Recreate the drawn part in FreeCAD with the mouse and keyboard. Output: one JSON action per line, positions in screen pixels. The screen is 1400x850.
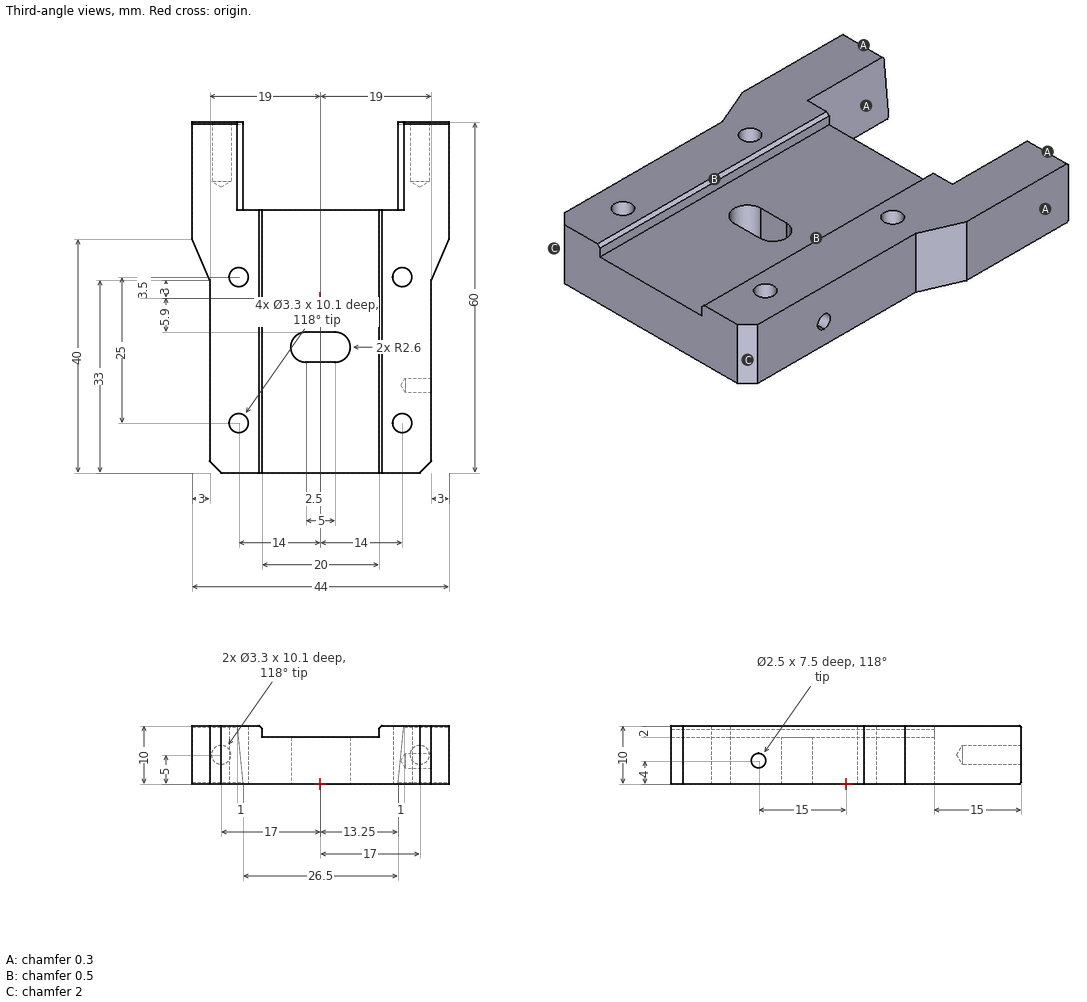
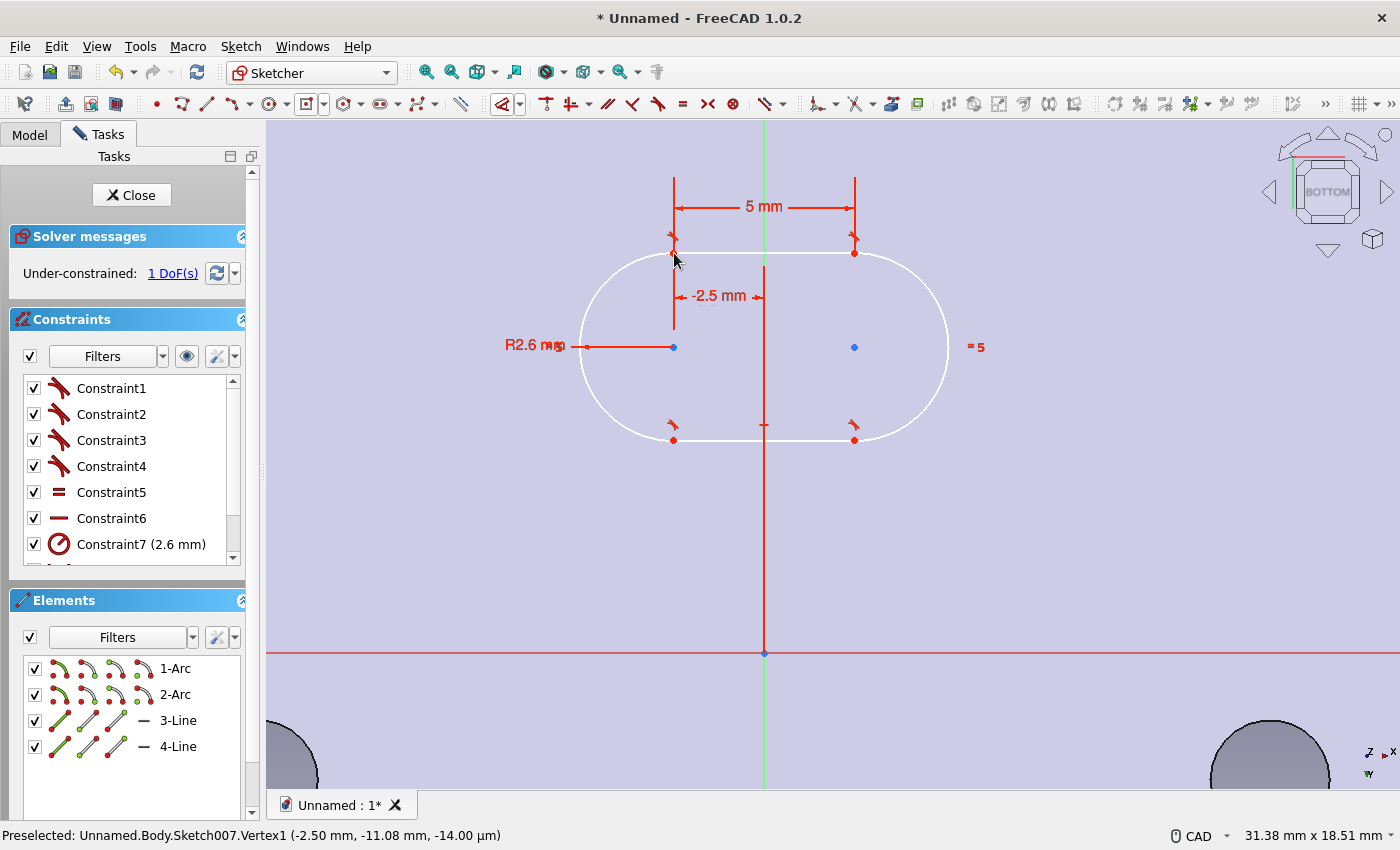
{"action": "left_click", "coordinate": [674, 441]}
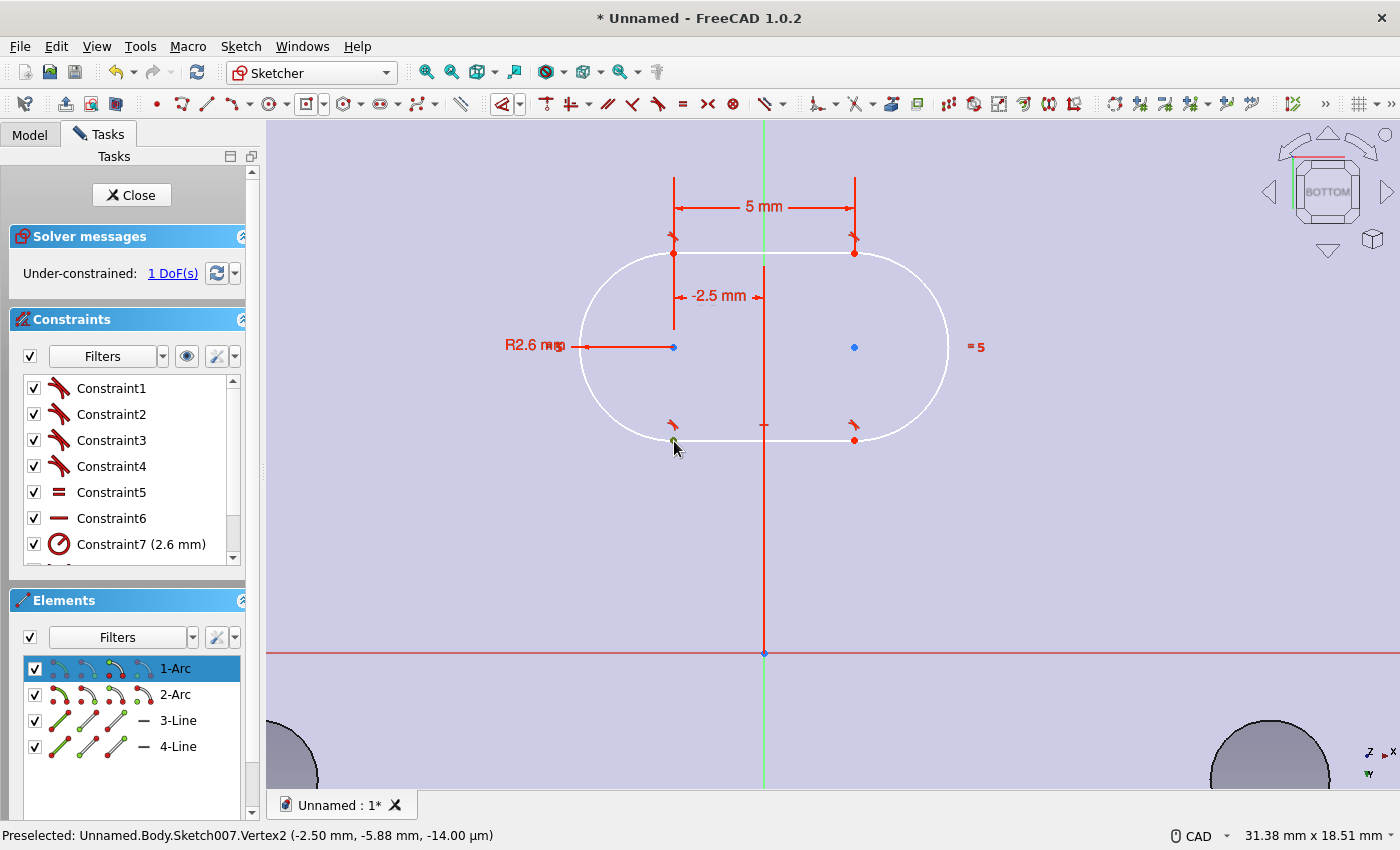
{"action": "left_click", "coordinate": [520, 104]}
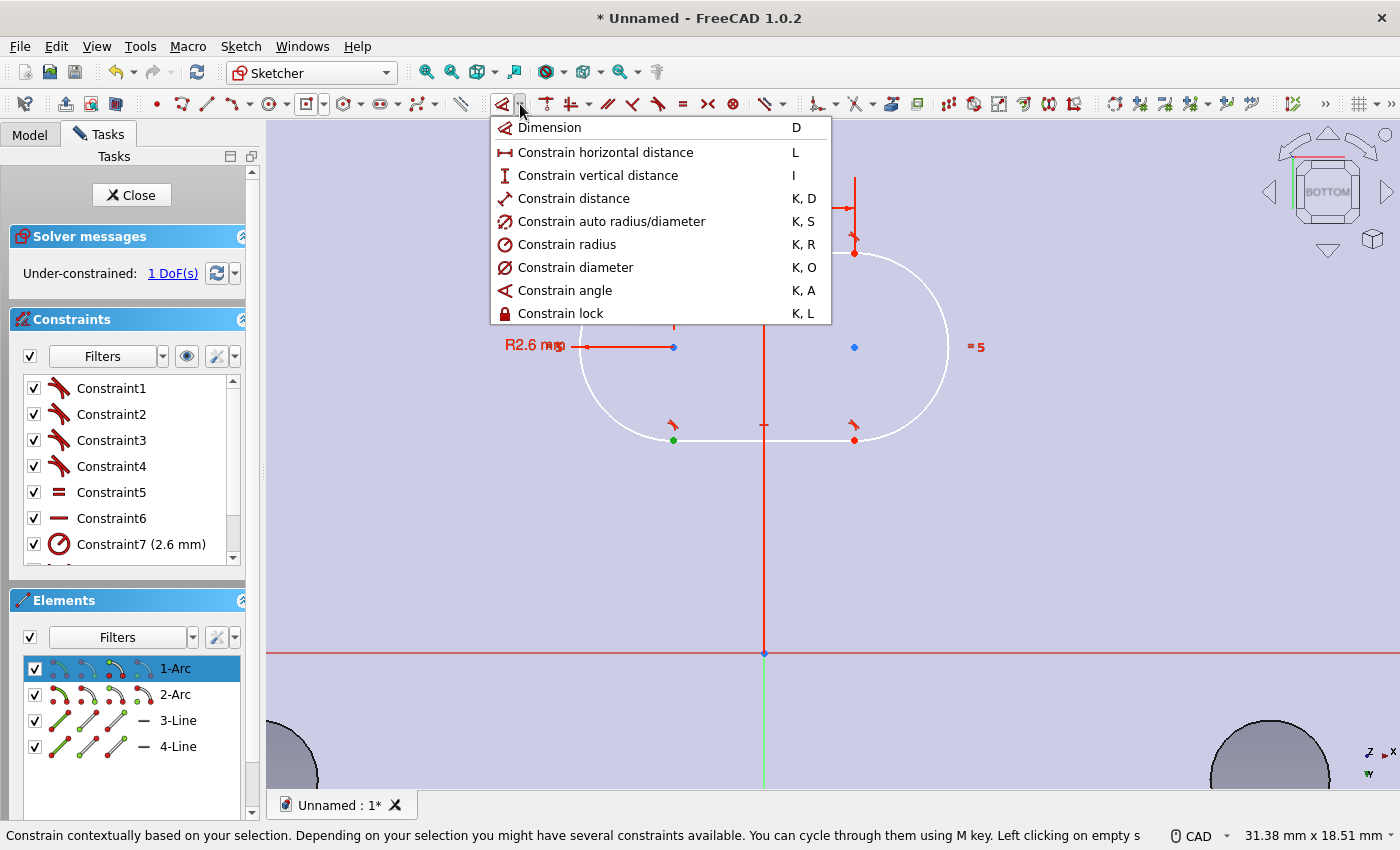
{"action": "left_click", "coordinate": [661, 176]}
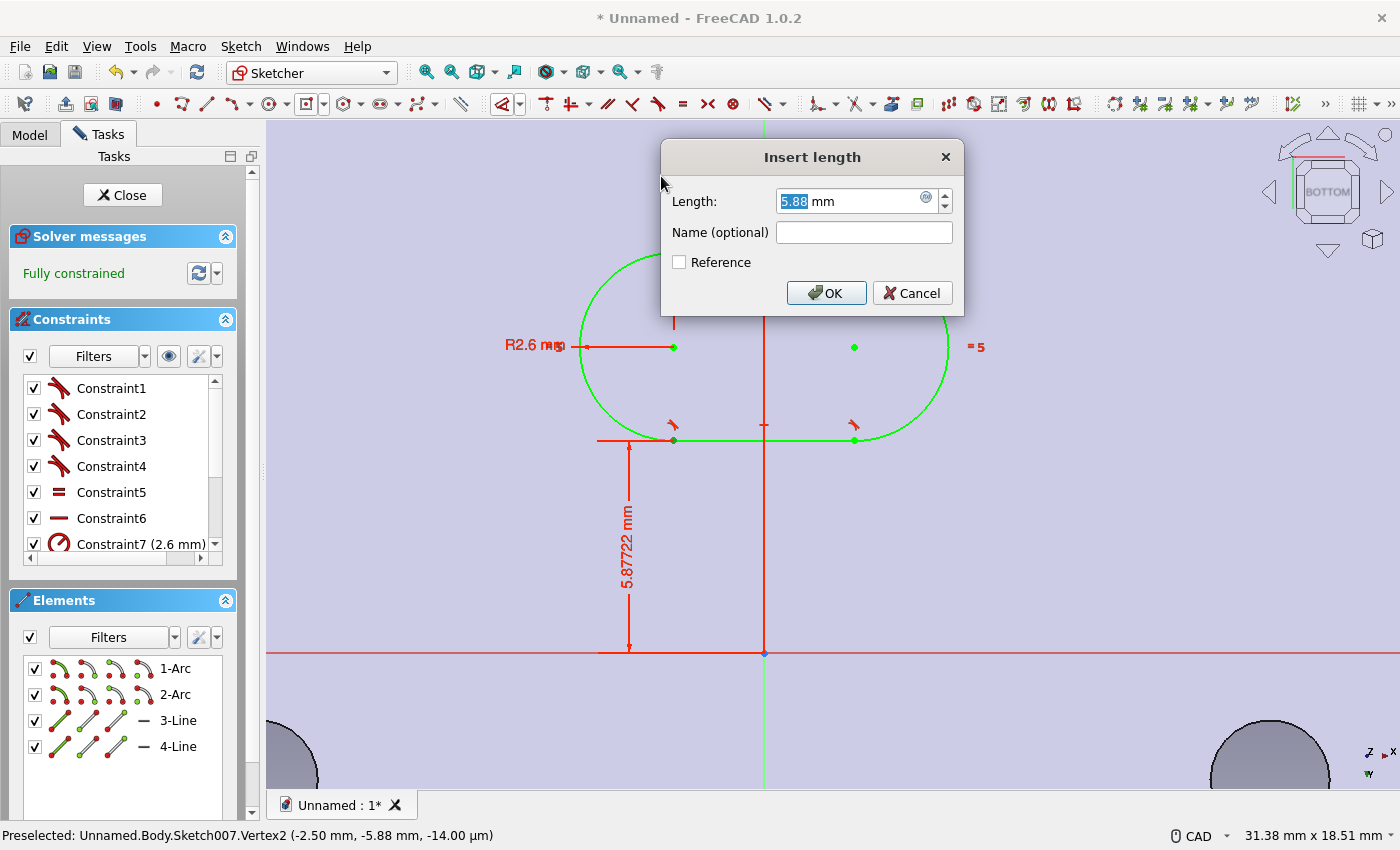
{"action": "type", "text": "5.9"}
{"action": "key", "text": "Return"}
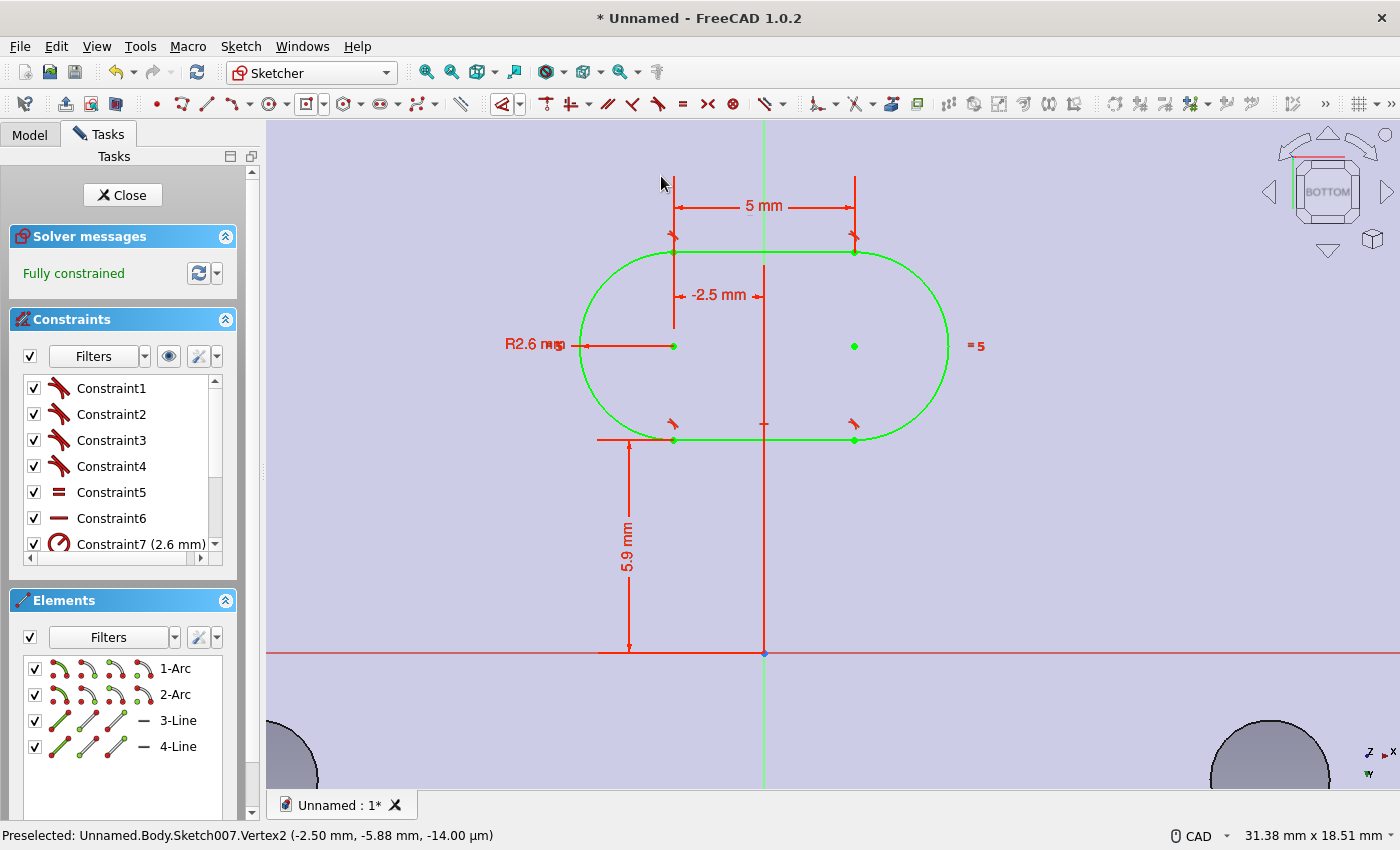
{"action": "left_click", "coordinate": [123, 195]}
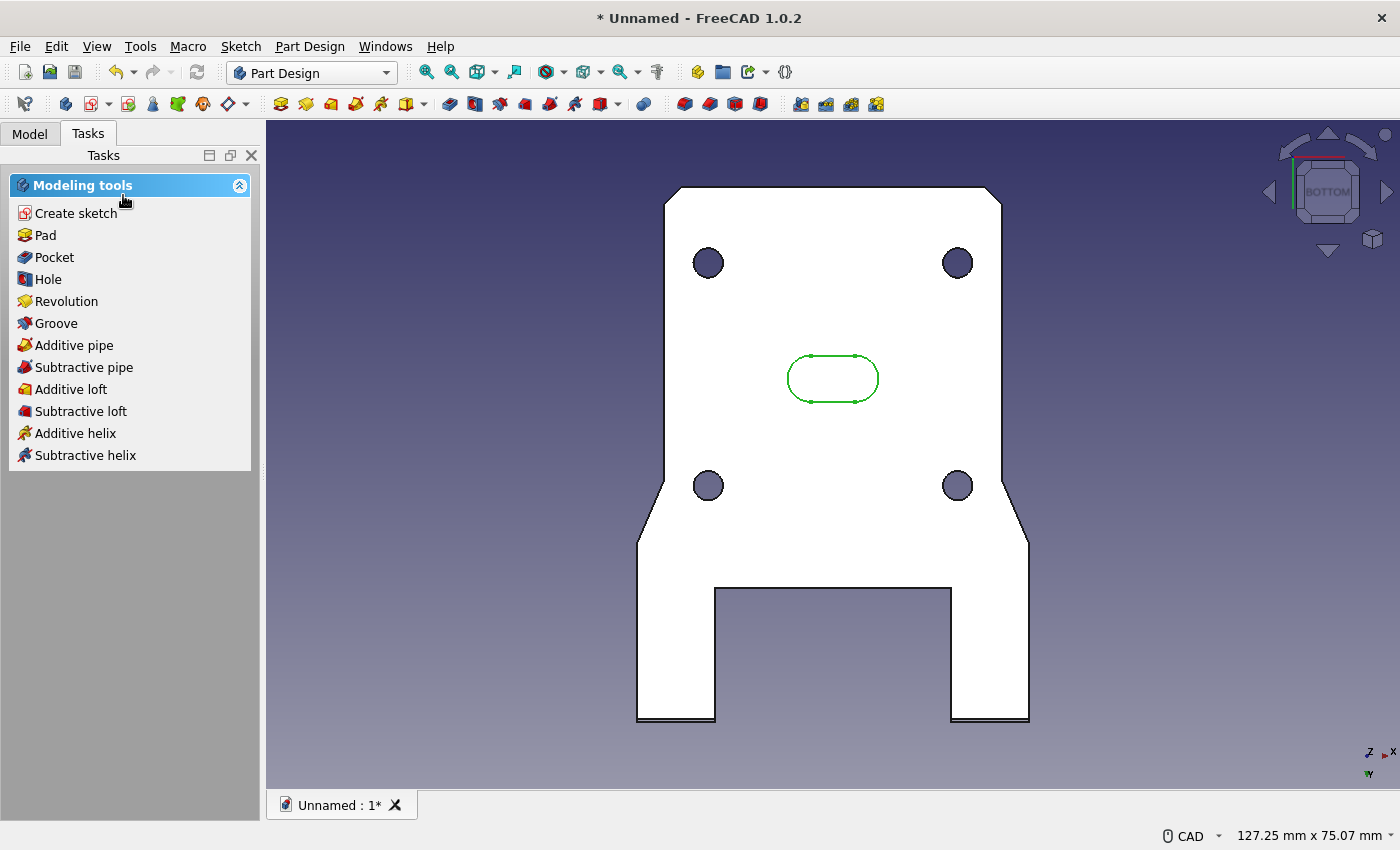
{"action": "left_click", "coordinate": [450, 104]}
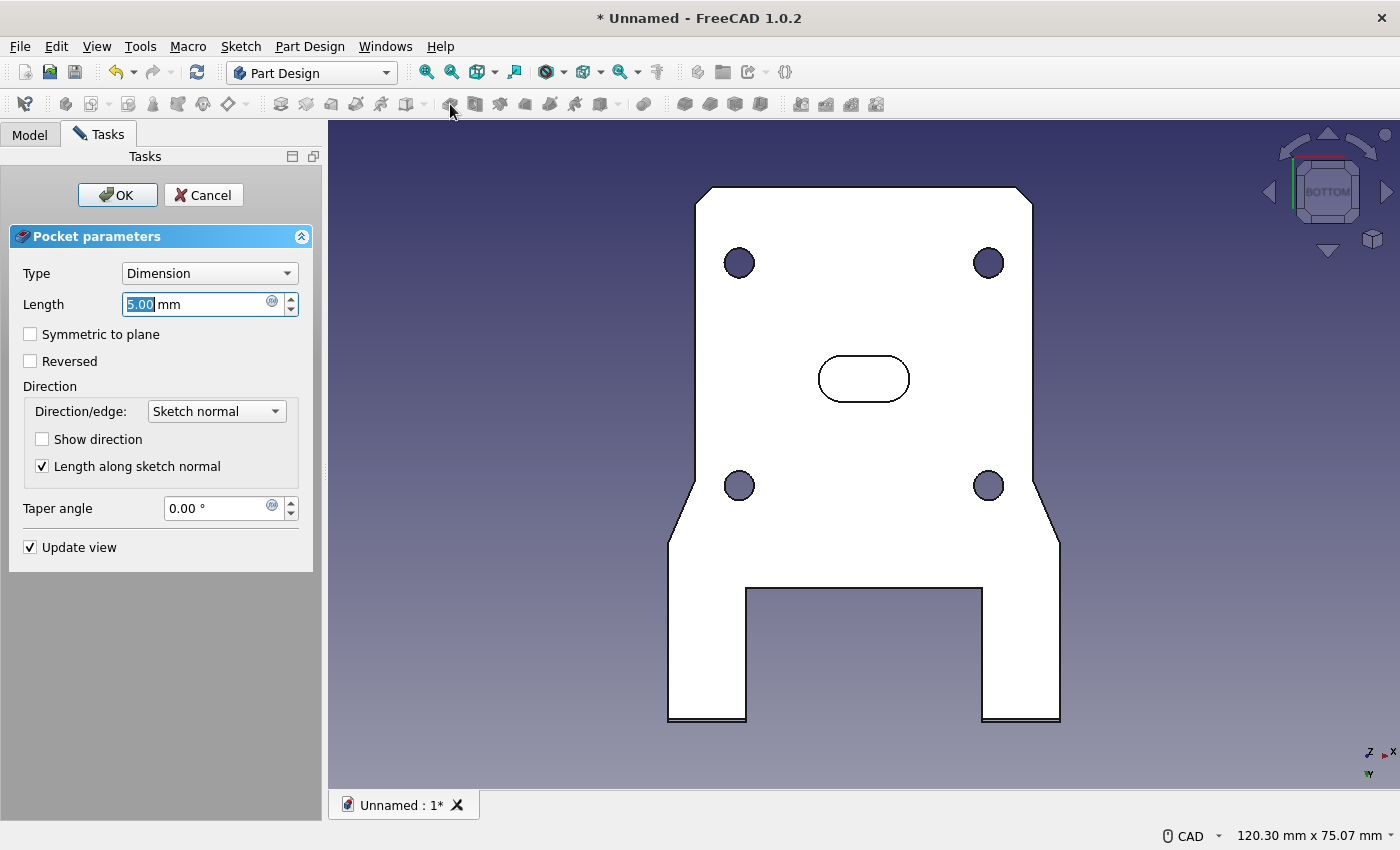
{"action": "left_click", "coordinate": [210, 274]}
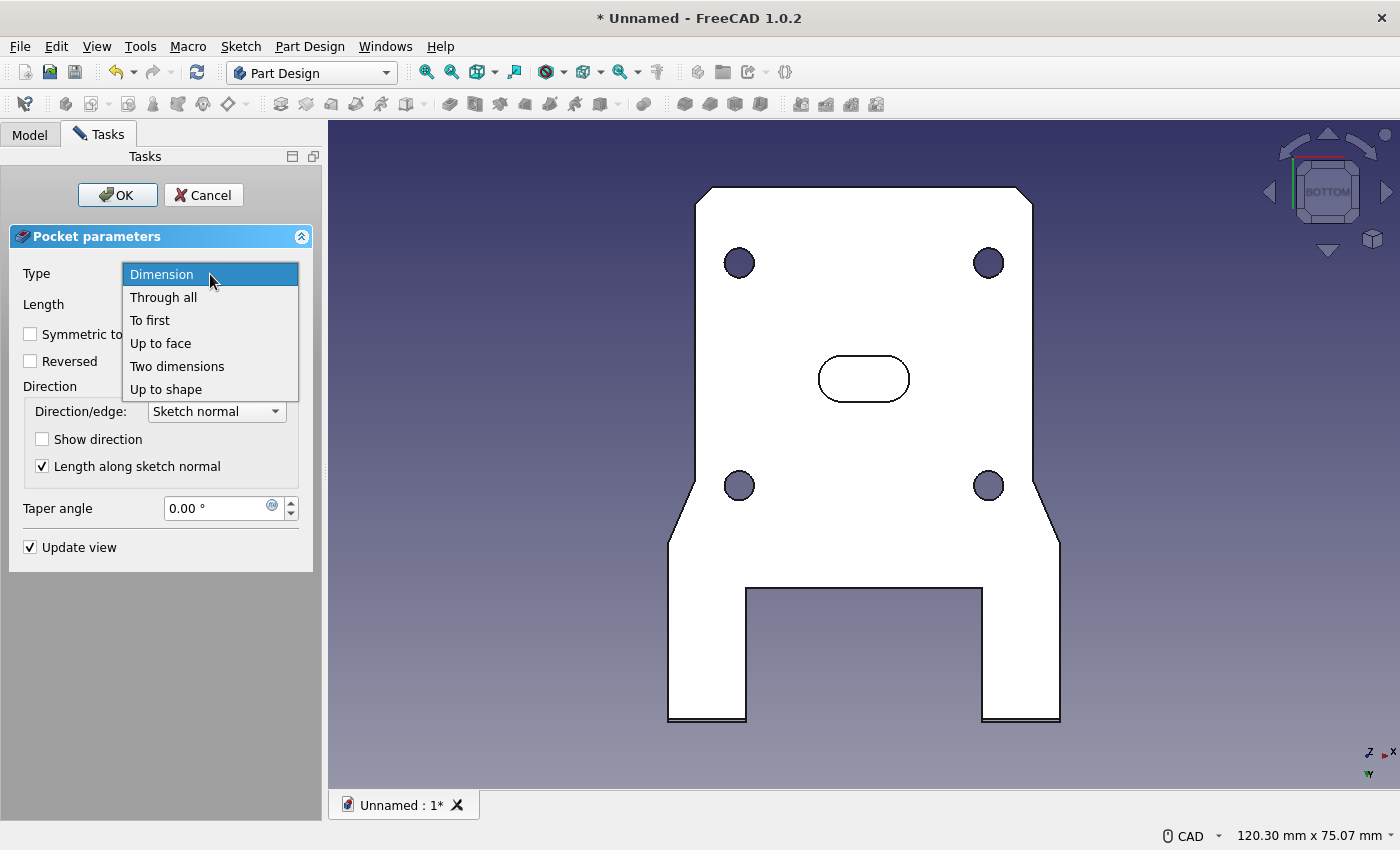
{"action": "left_click", "coordinate": [208, 298]}